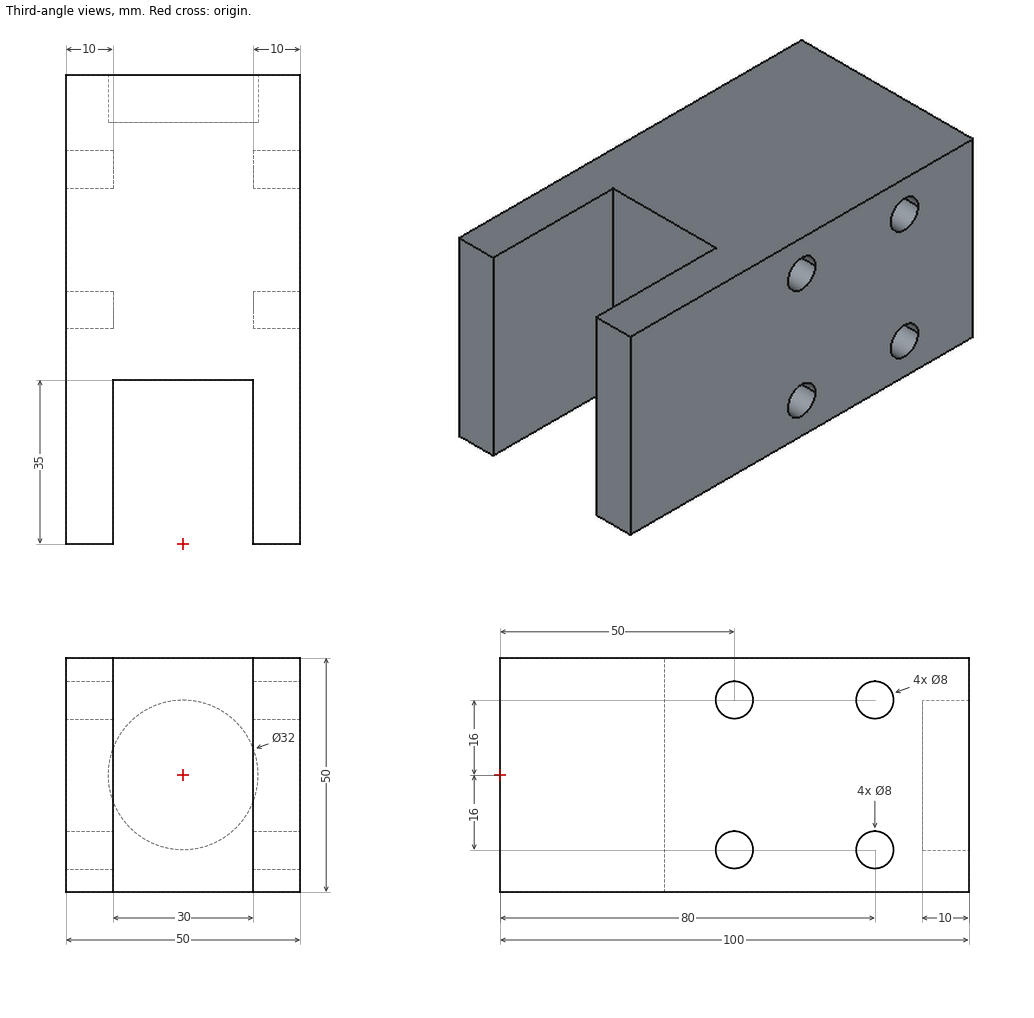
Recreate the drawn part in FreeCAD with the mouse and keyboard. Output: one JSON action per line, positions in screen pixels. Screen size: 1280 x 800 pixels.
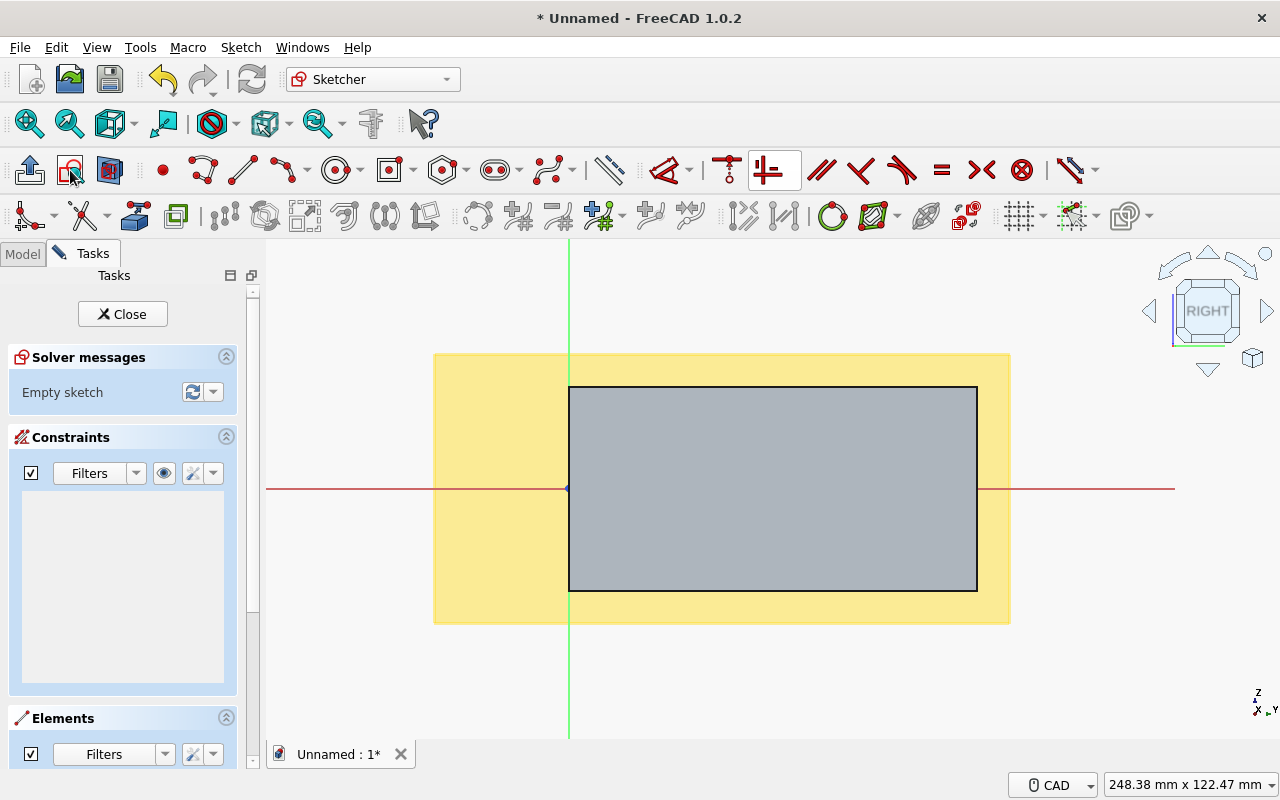
{"action": "left_click", "coordinate": [110, 170]}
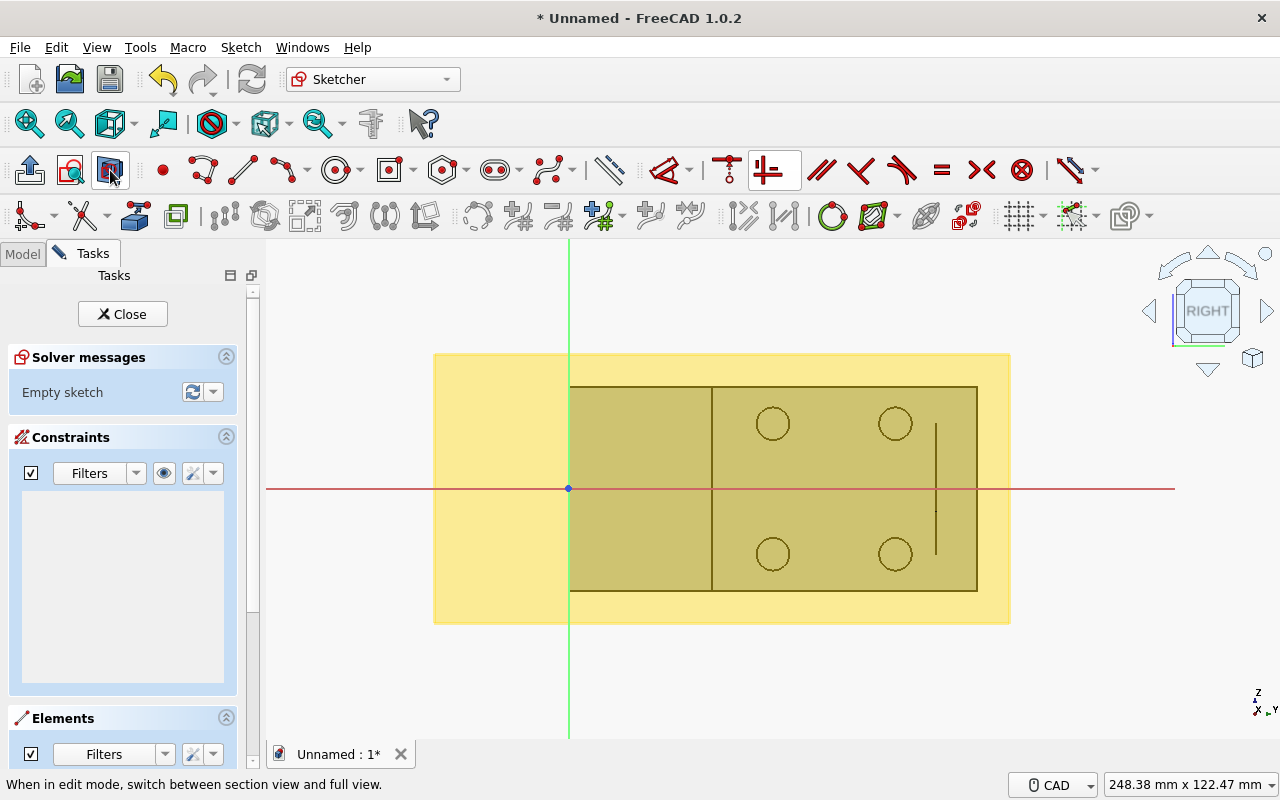
{"action": "scroll", "coordinate": [784, 489], "scroll_direction": "up", "scroll_amount": 3}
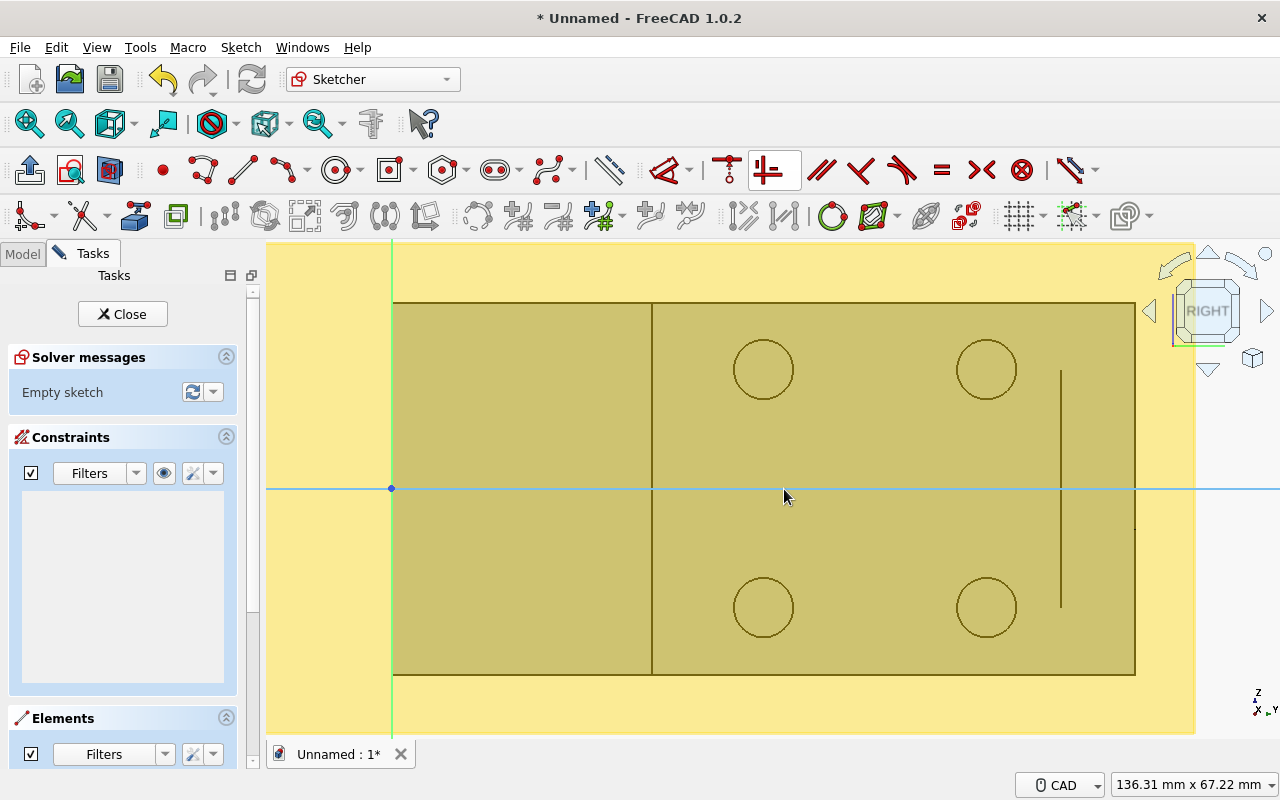
{"action": "left_click", "coordinate": [336, 170]}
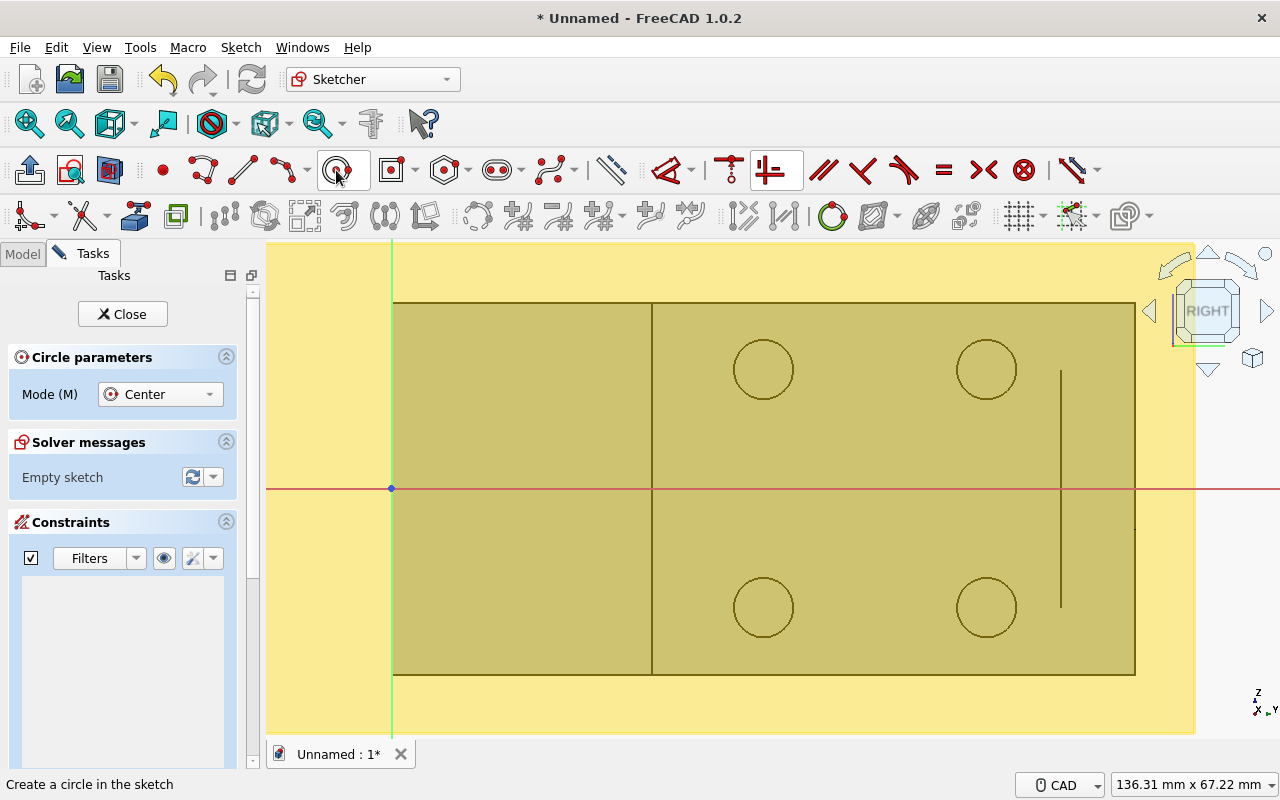
{"action": "left_click", "coordinate": [987, 370]}
{"action": "mouse_move", "coordinate": [1008, 349]}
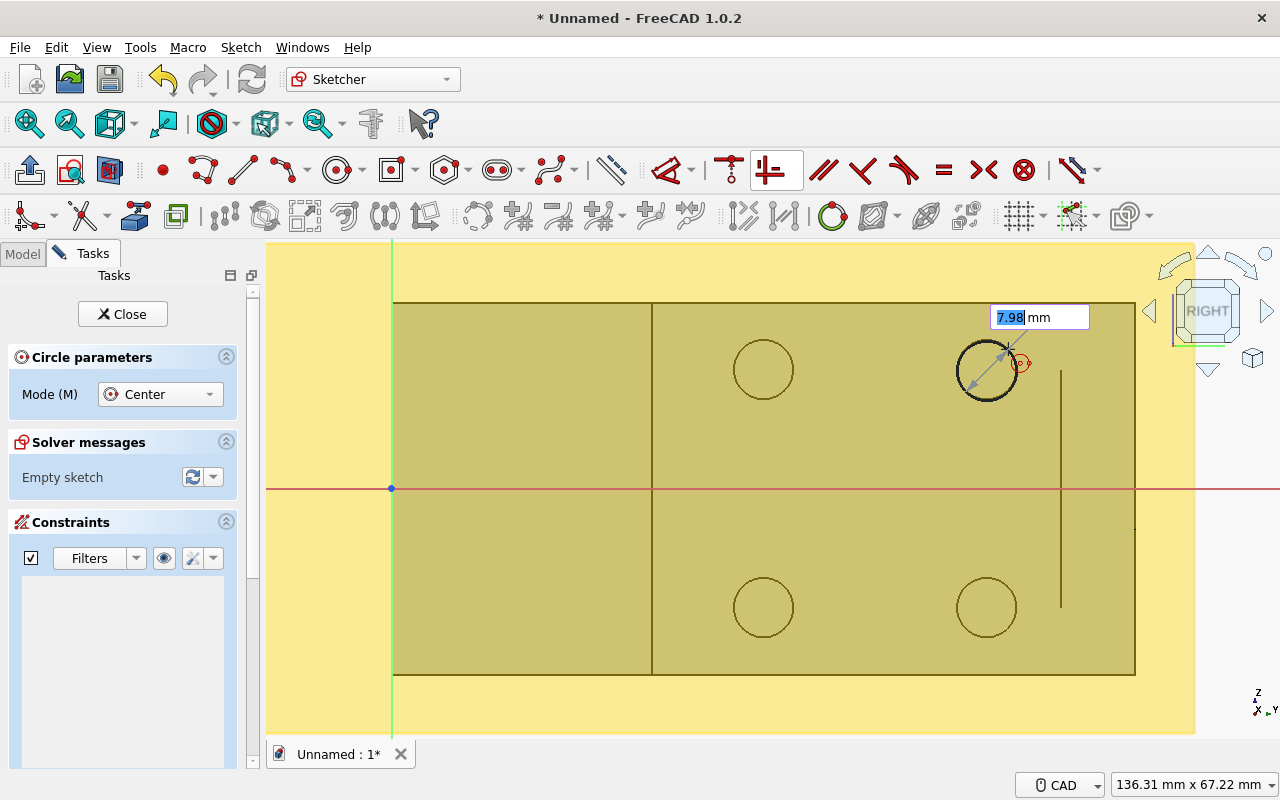
{"action": "type", "text": "8"}
{"action": "key", "text": "Return"}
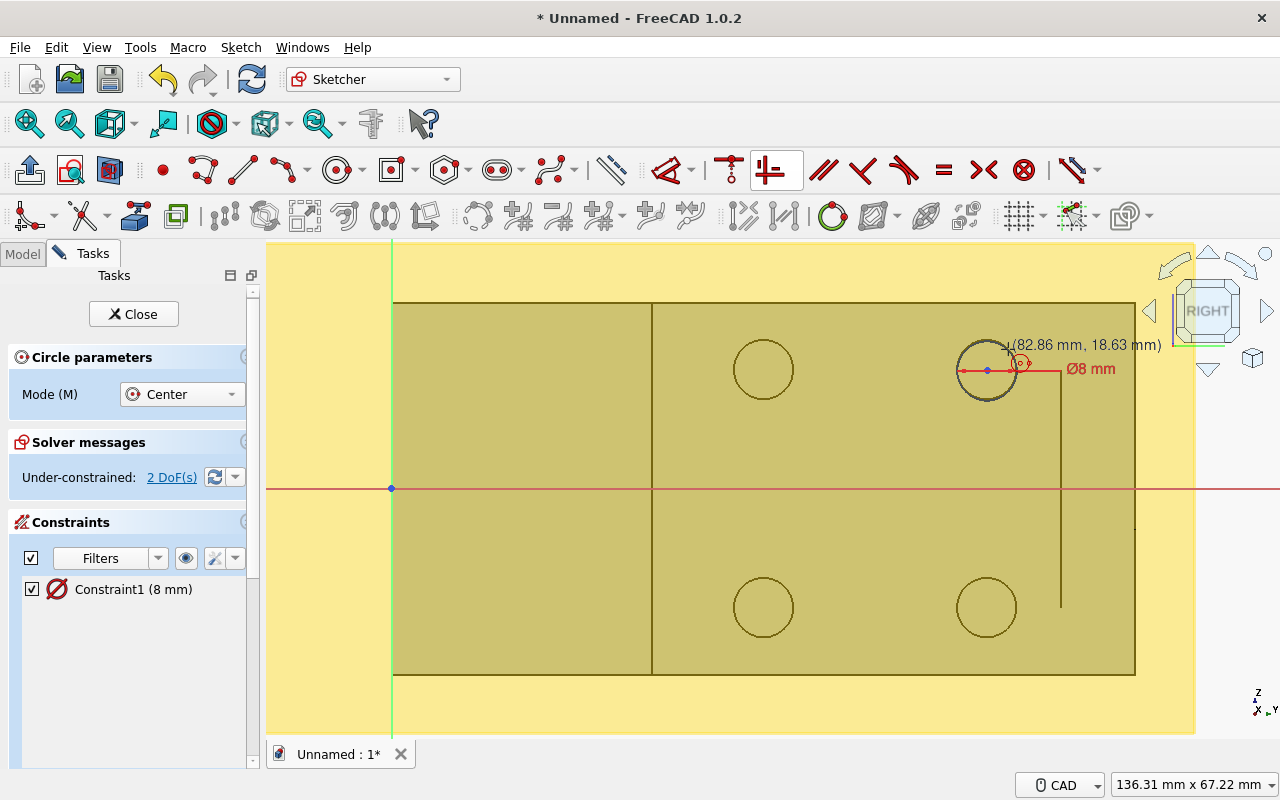
{"action": "left_click", "coordinate": [764, 370]}
{"action": "mouse_move", "coordinate": [785, 349]}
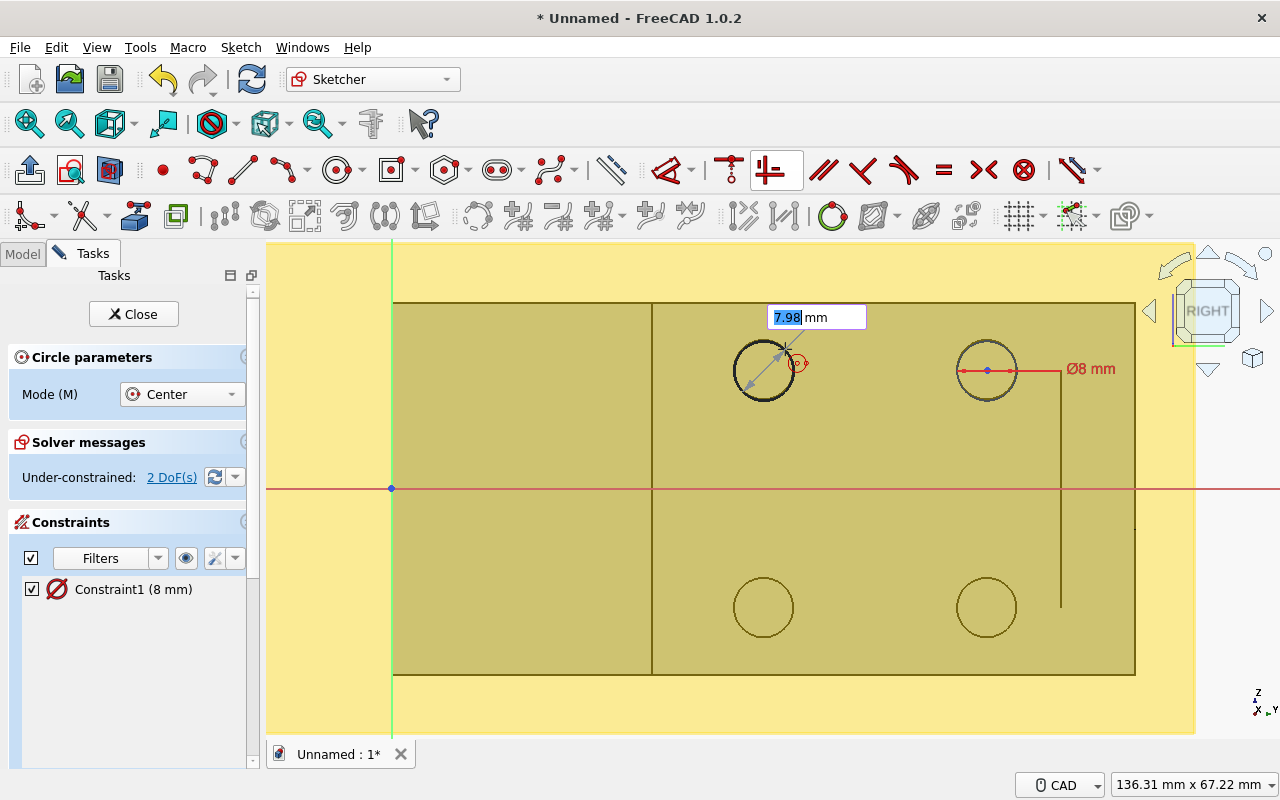
{"action": "type", "text": "8"}
{"action": "key", "text": "Return"}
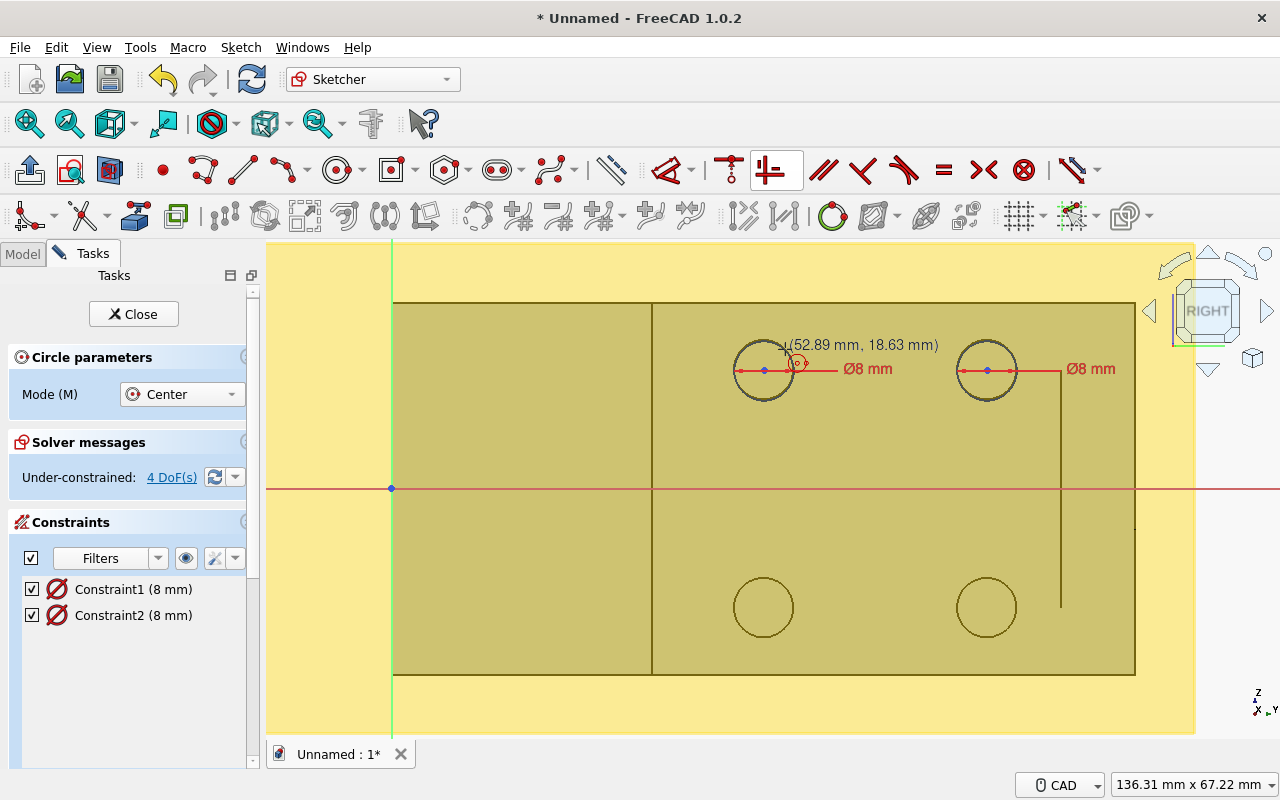
{"action": "left_click", "coordinate": [764, 608]}
{"action": "mouse_move", "coordinate": [785, 587]}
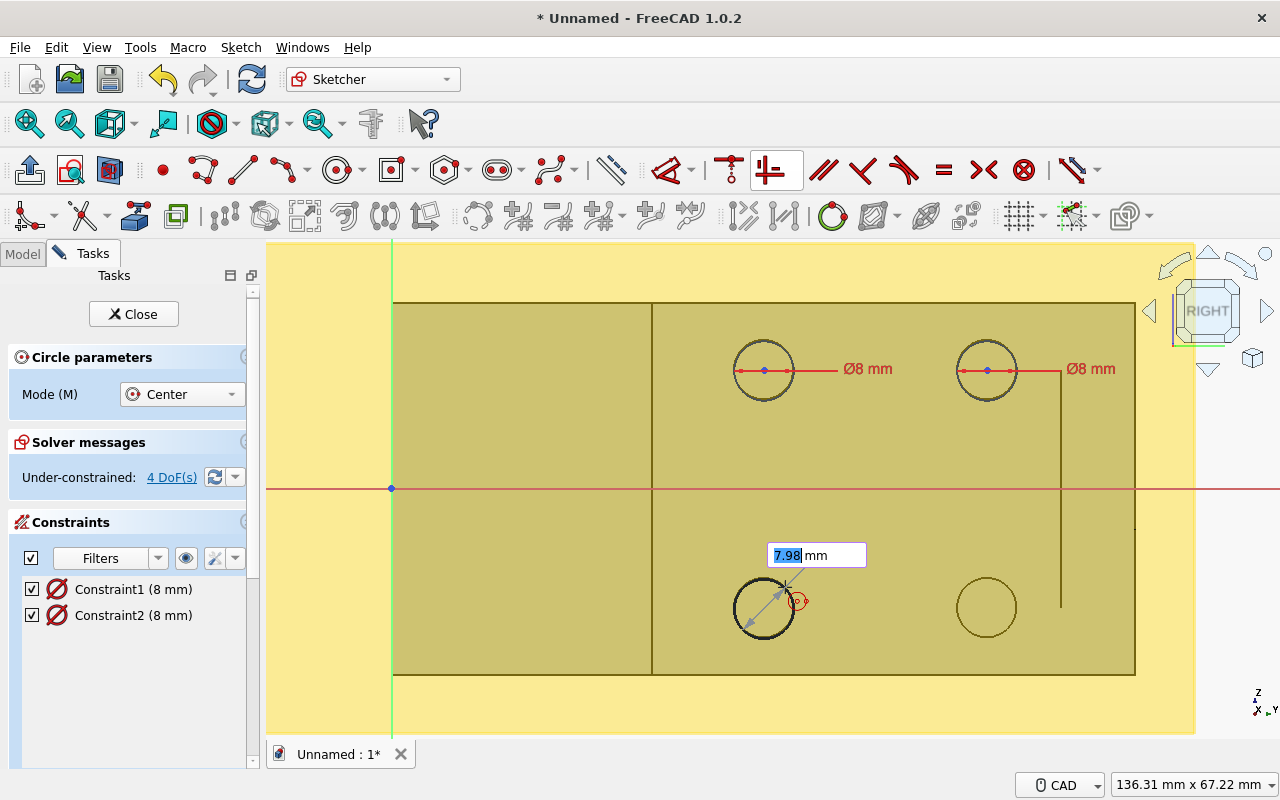
{"action": "type", "text": "8"}
{"action": "key", "text": "Return"}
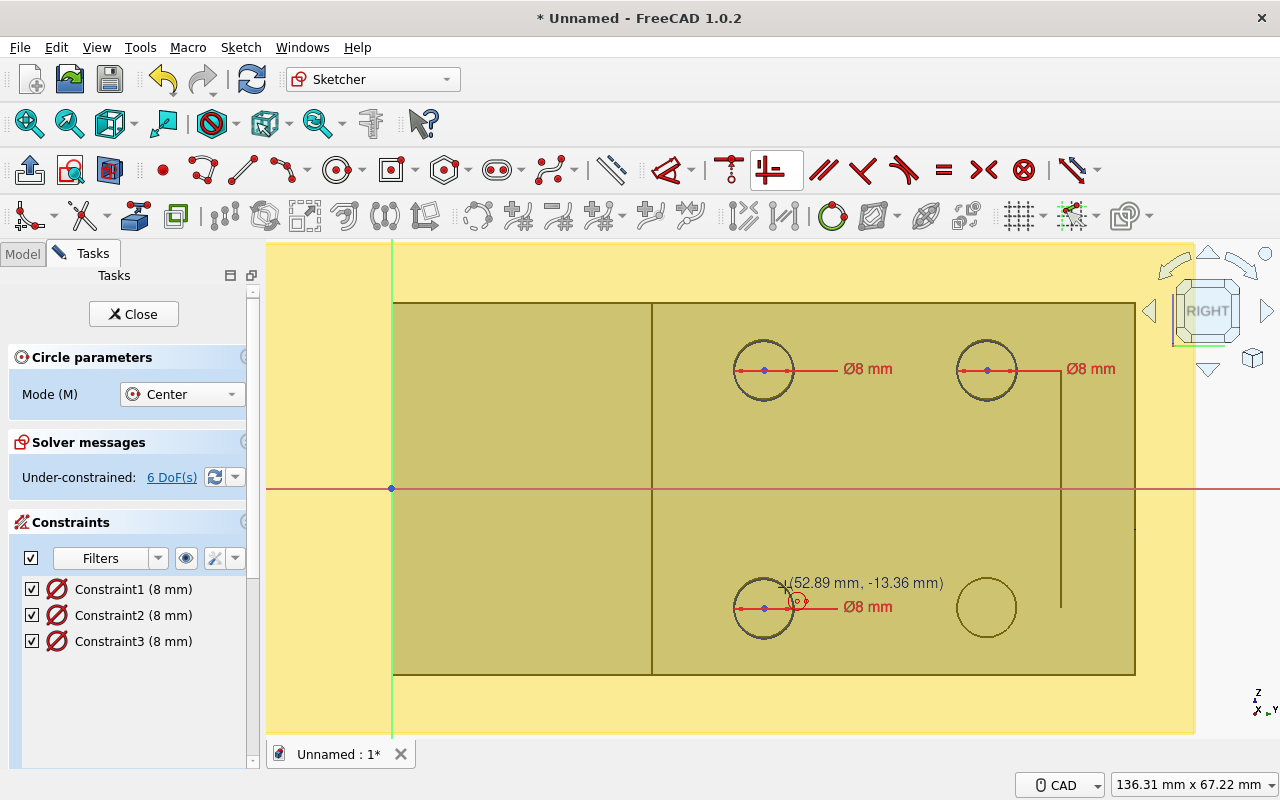
{"action": "left_click", "coordinate": [987, 608]}
{"action": "mouse_move", "coordinate": [1008, 587]}